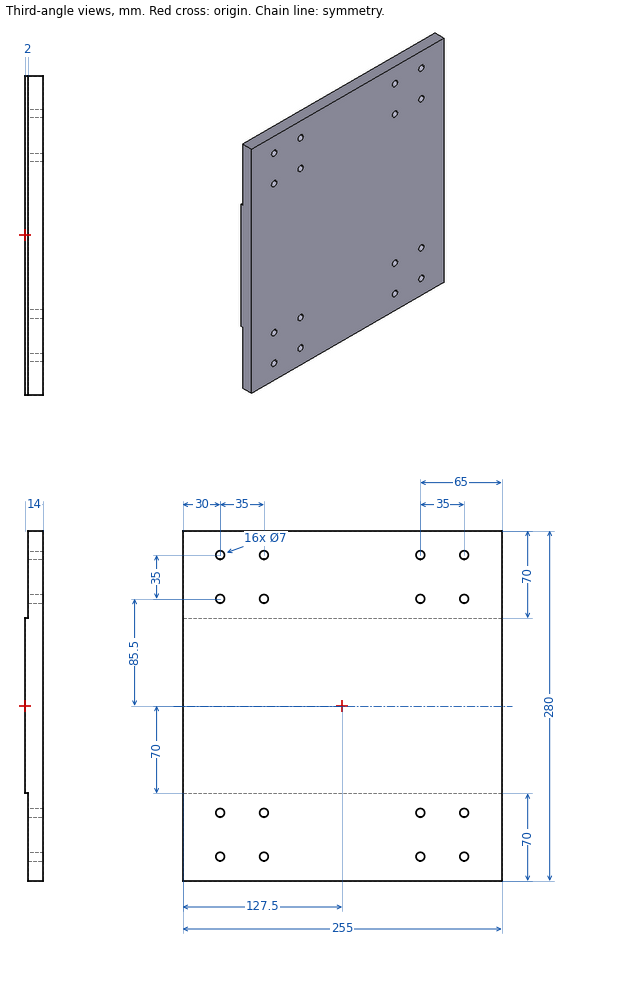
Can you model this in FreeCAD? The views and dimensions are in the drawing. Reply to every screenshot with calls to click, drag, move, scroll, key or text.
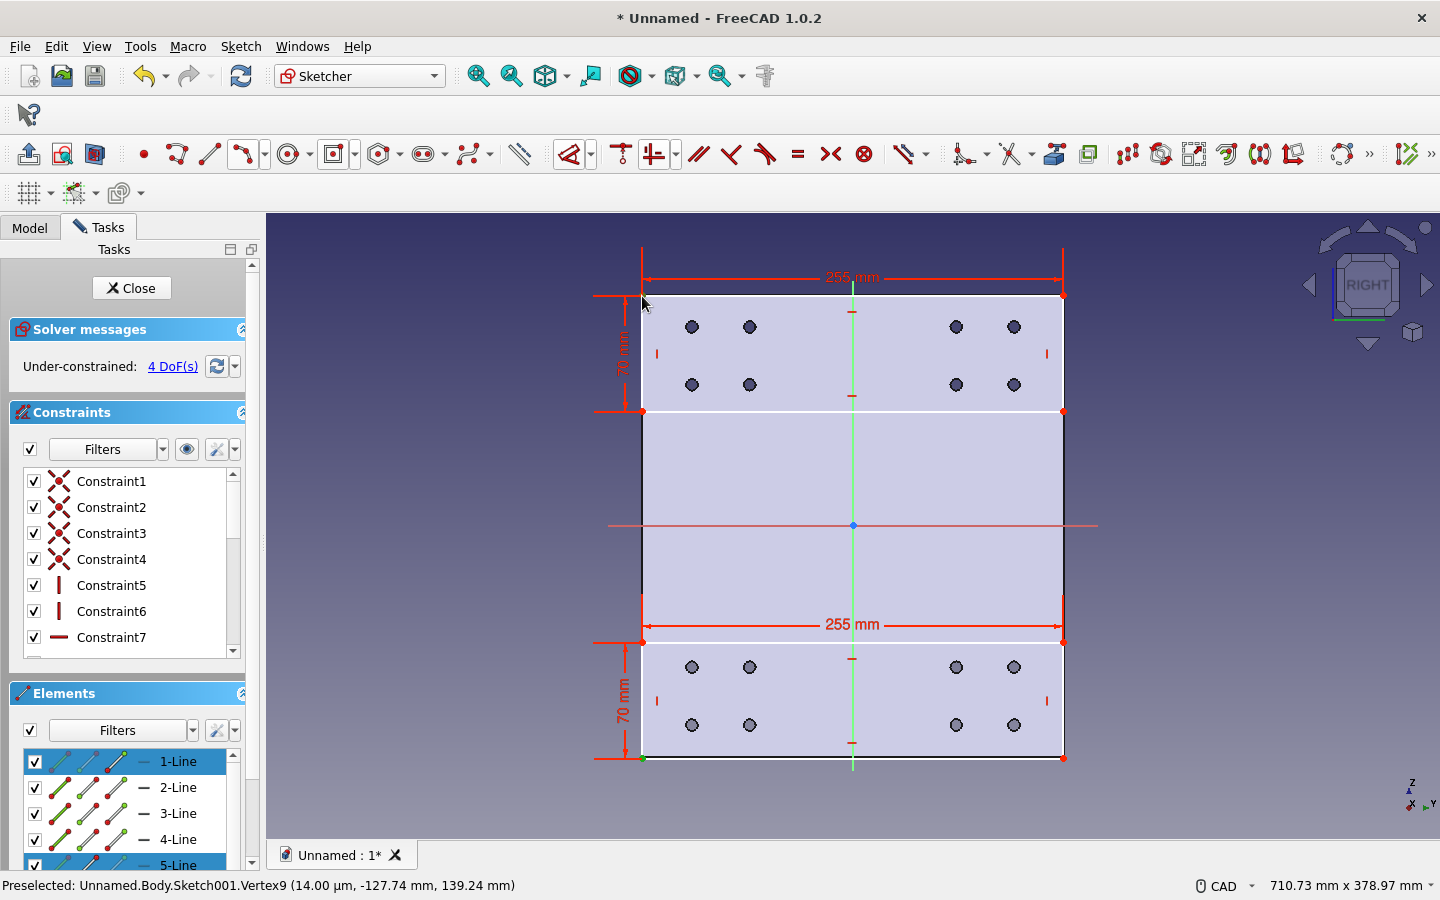
click(644, 526)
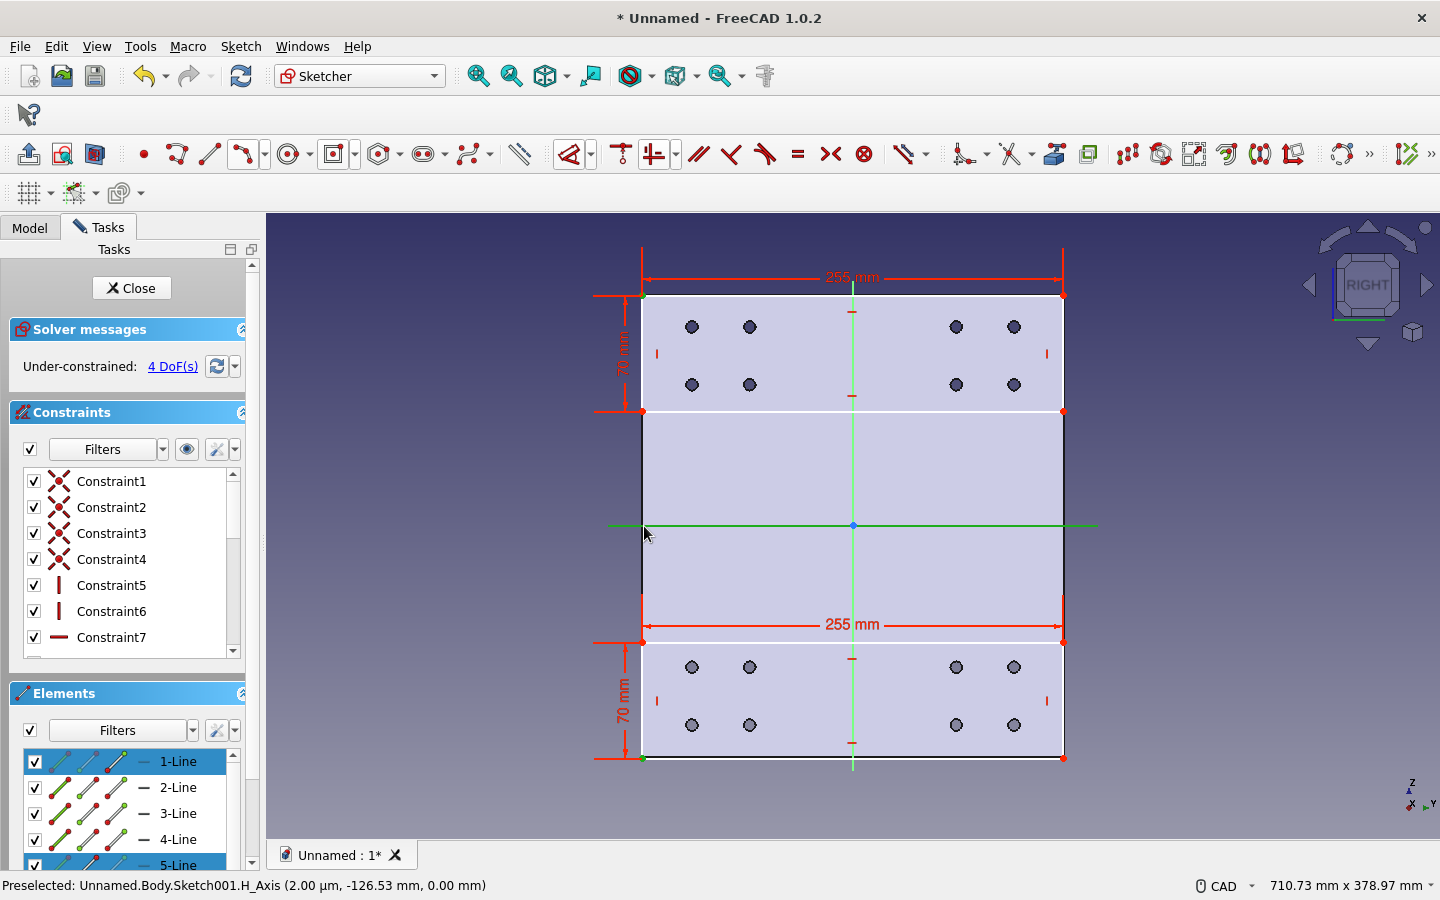
click(831, 154)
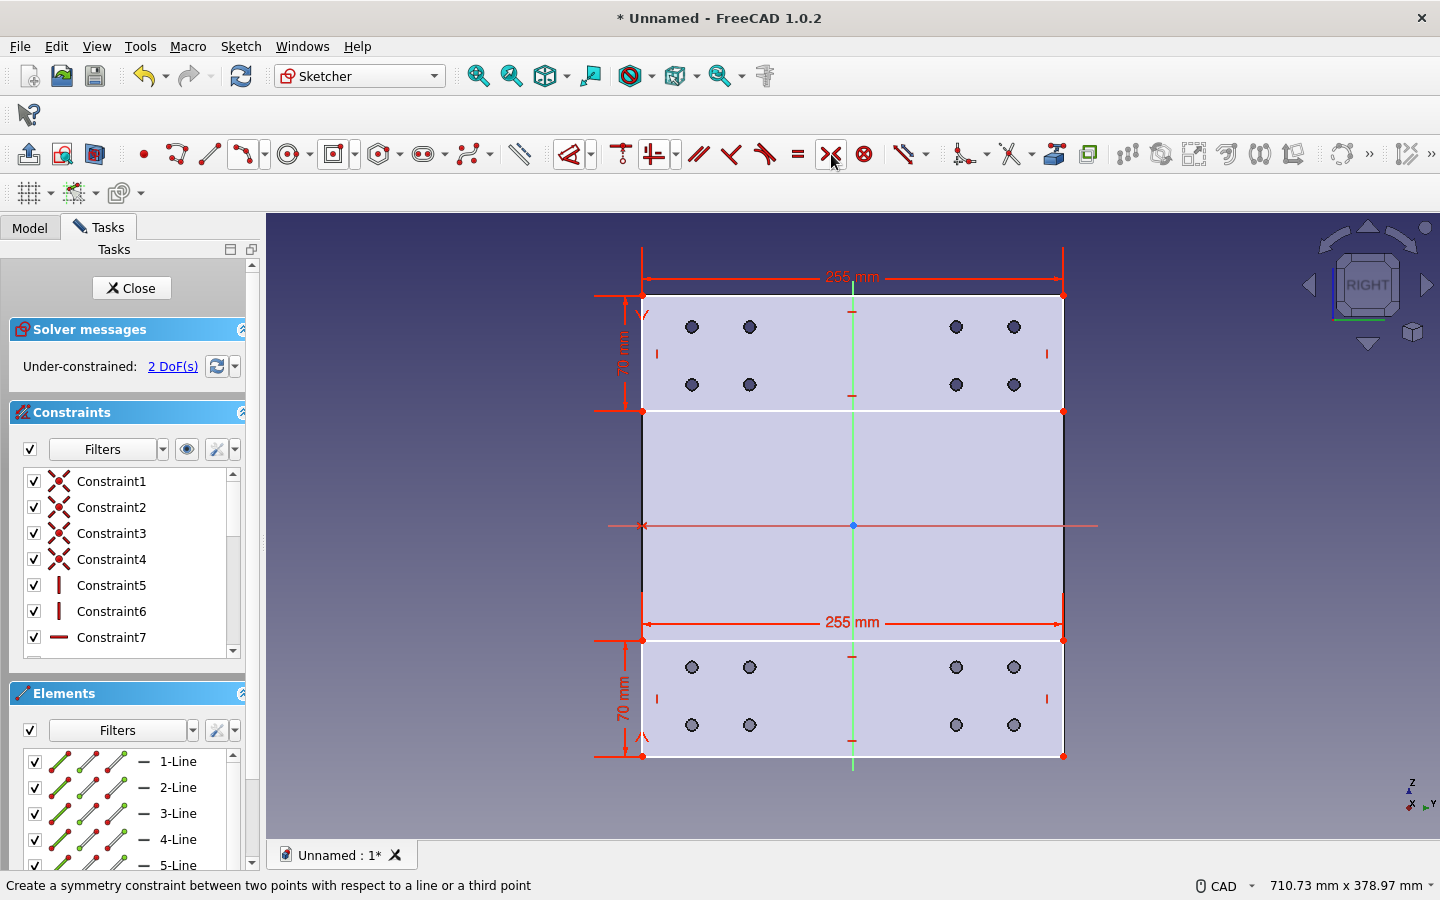
click(642, 641)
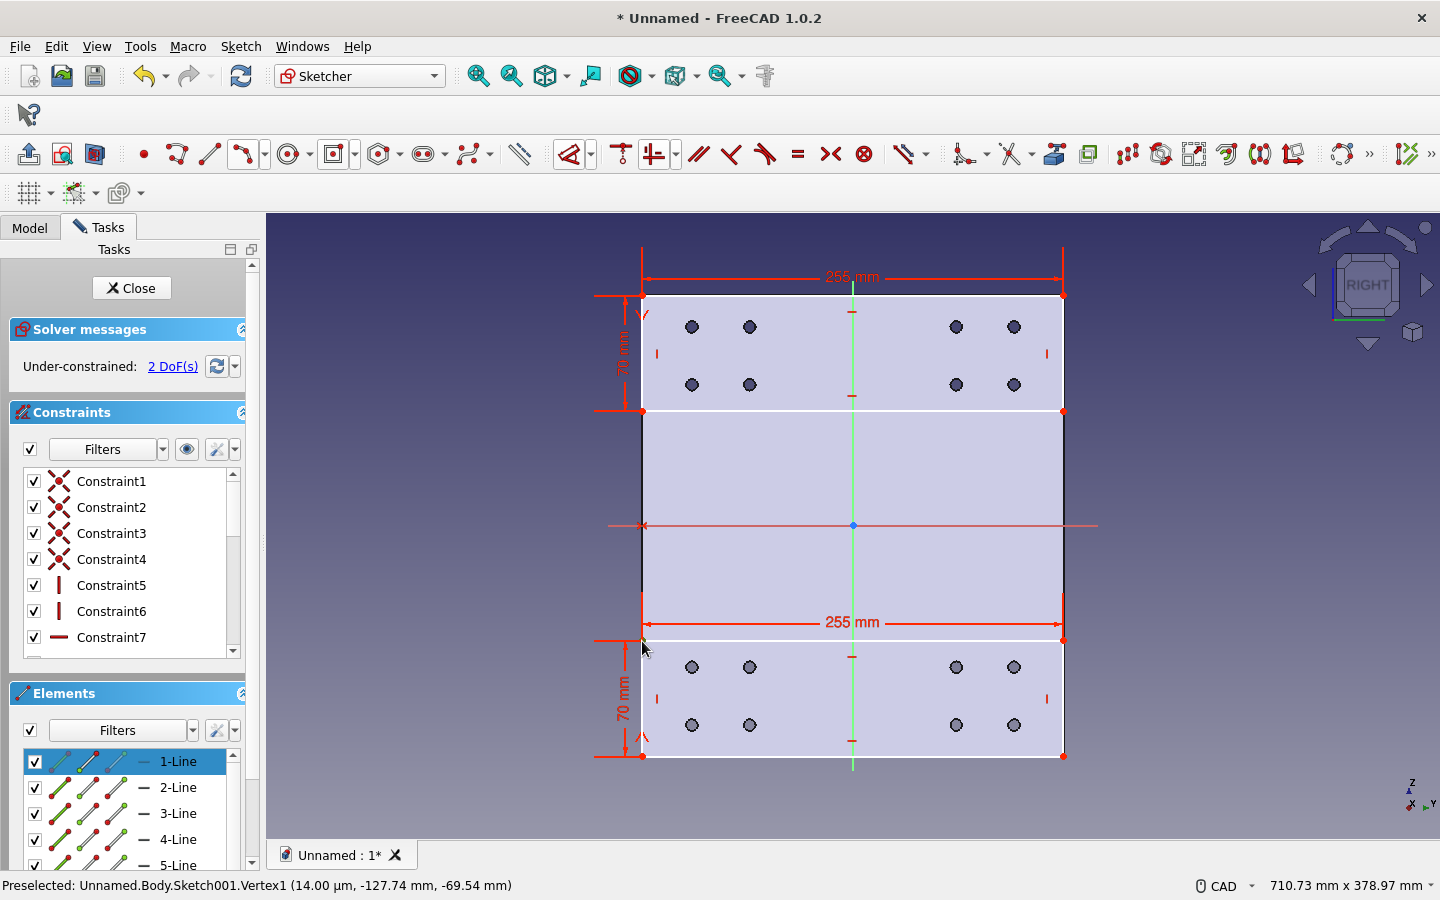
click(590, 154)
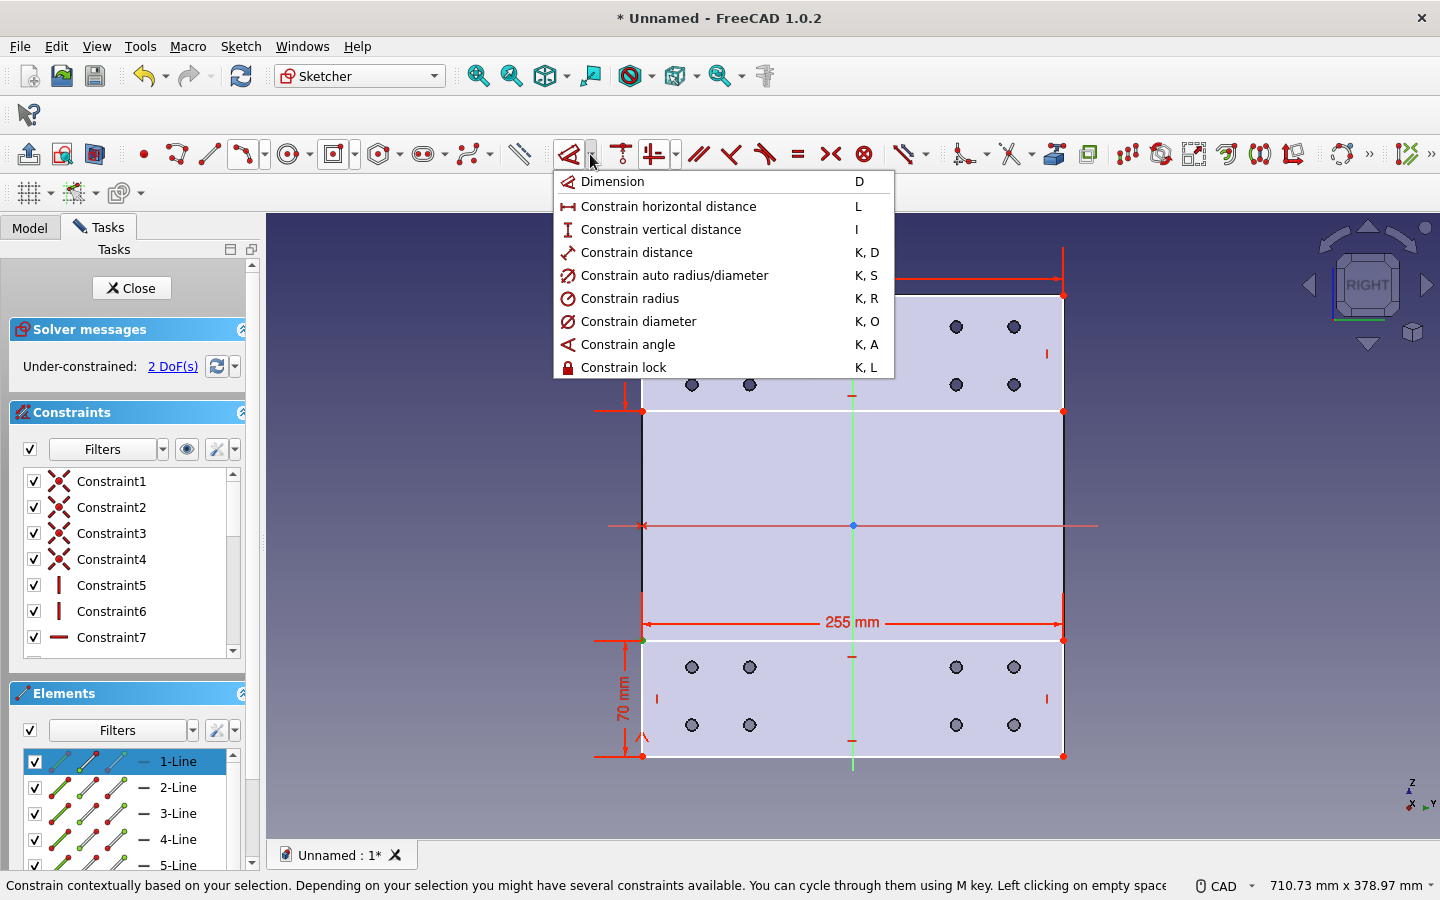
click(724, 230)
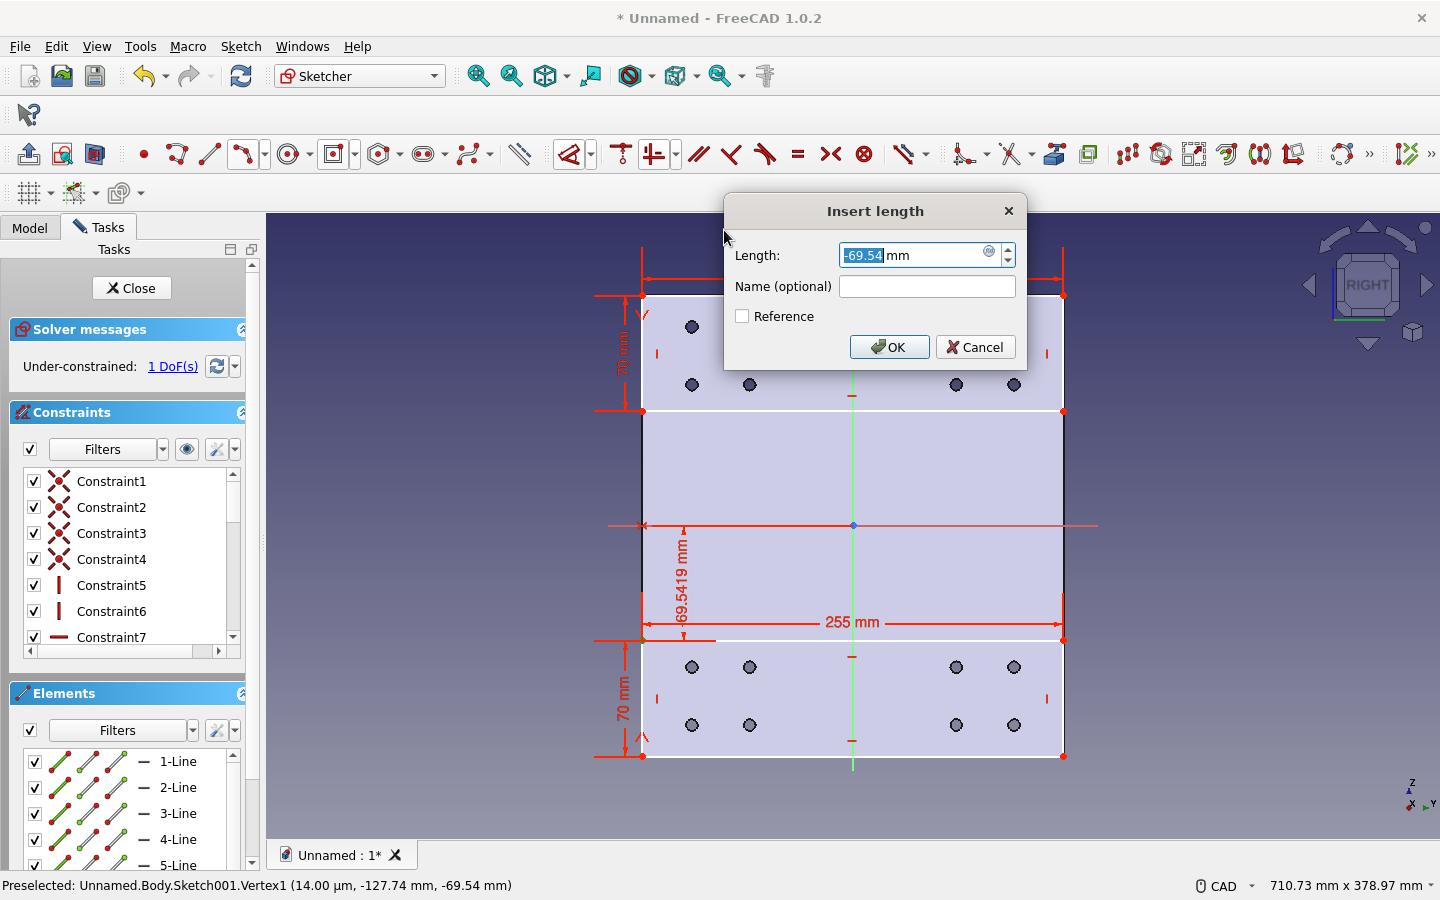
text(-70)
key(Return)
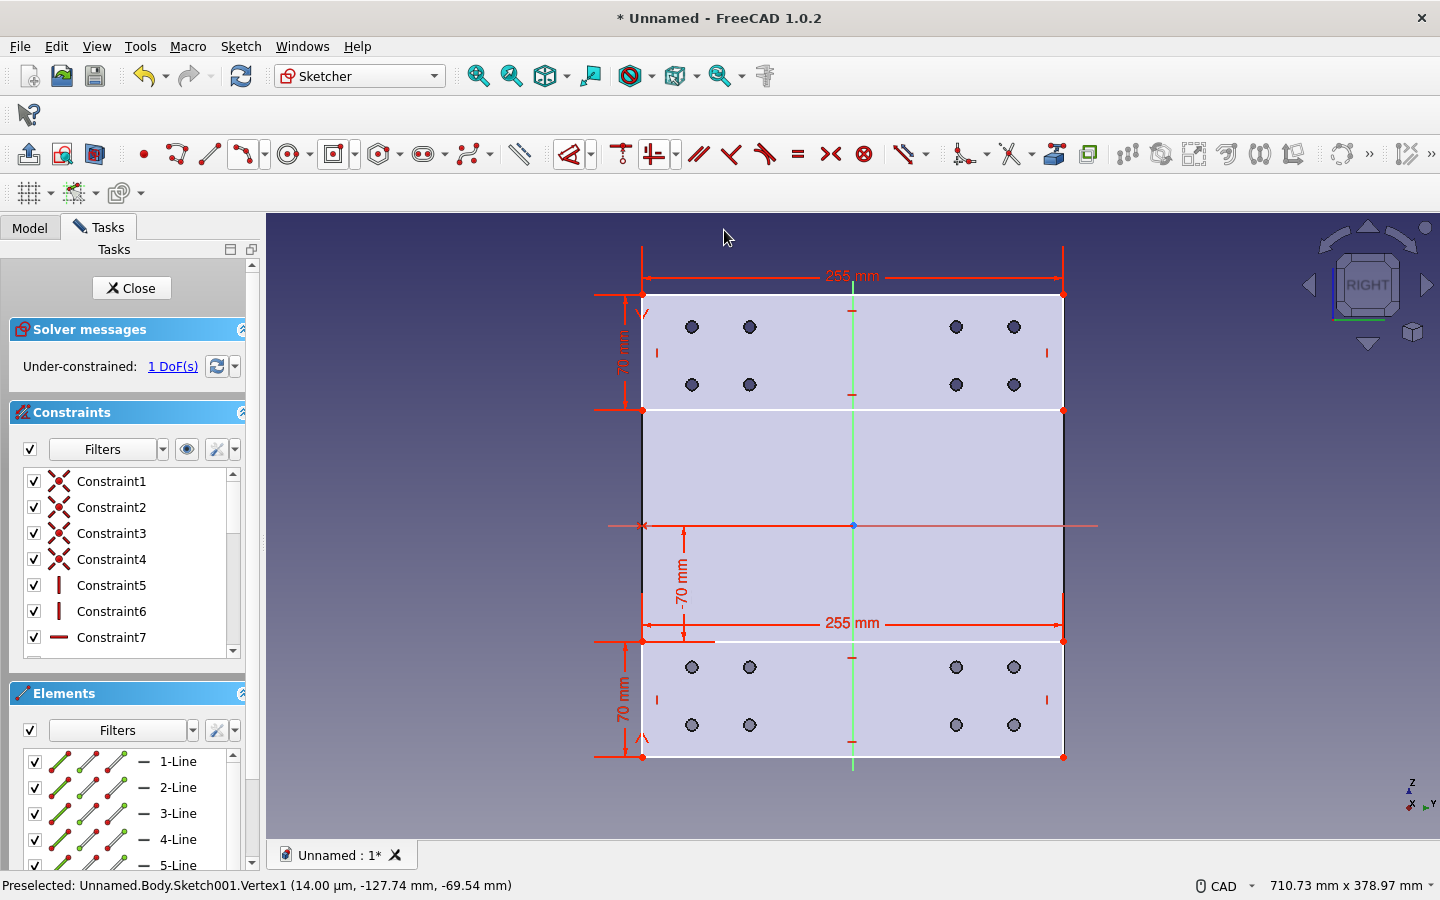
click(642, 642)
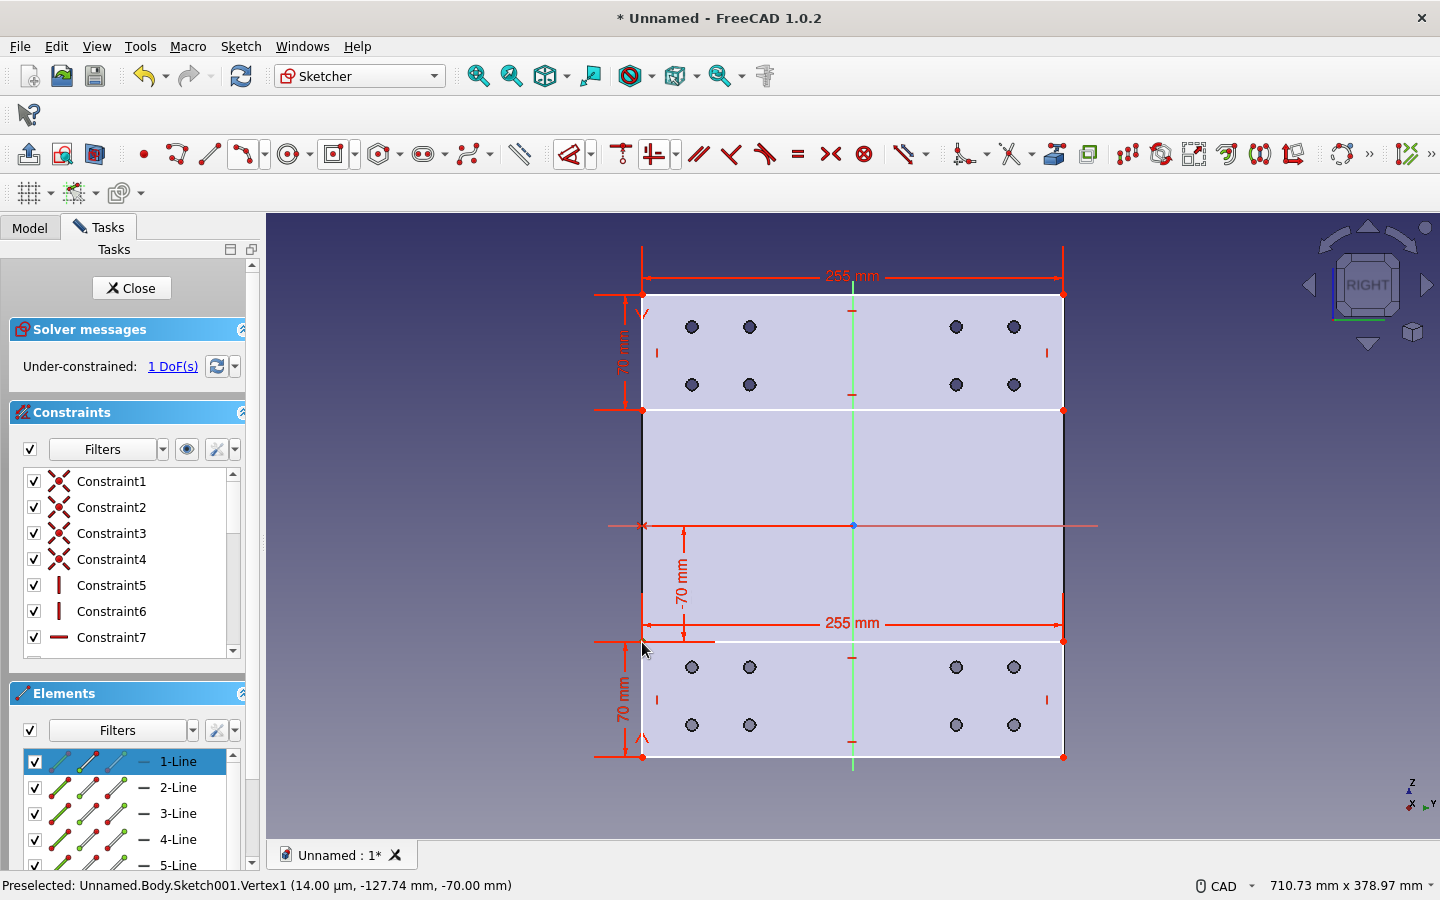
key(l)